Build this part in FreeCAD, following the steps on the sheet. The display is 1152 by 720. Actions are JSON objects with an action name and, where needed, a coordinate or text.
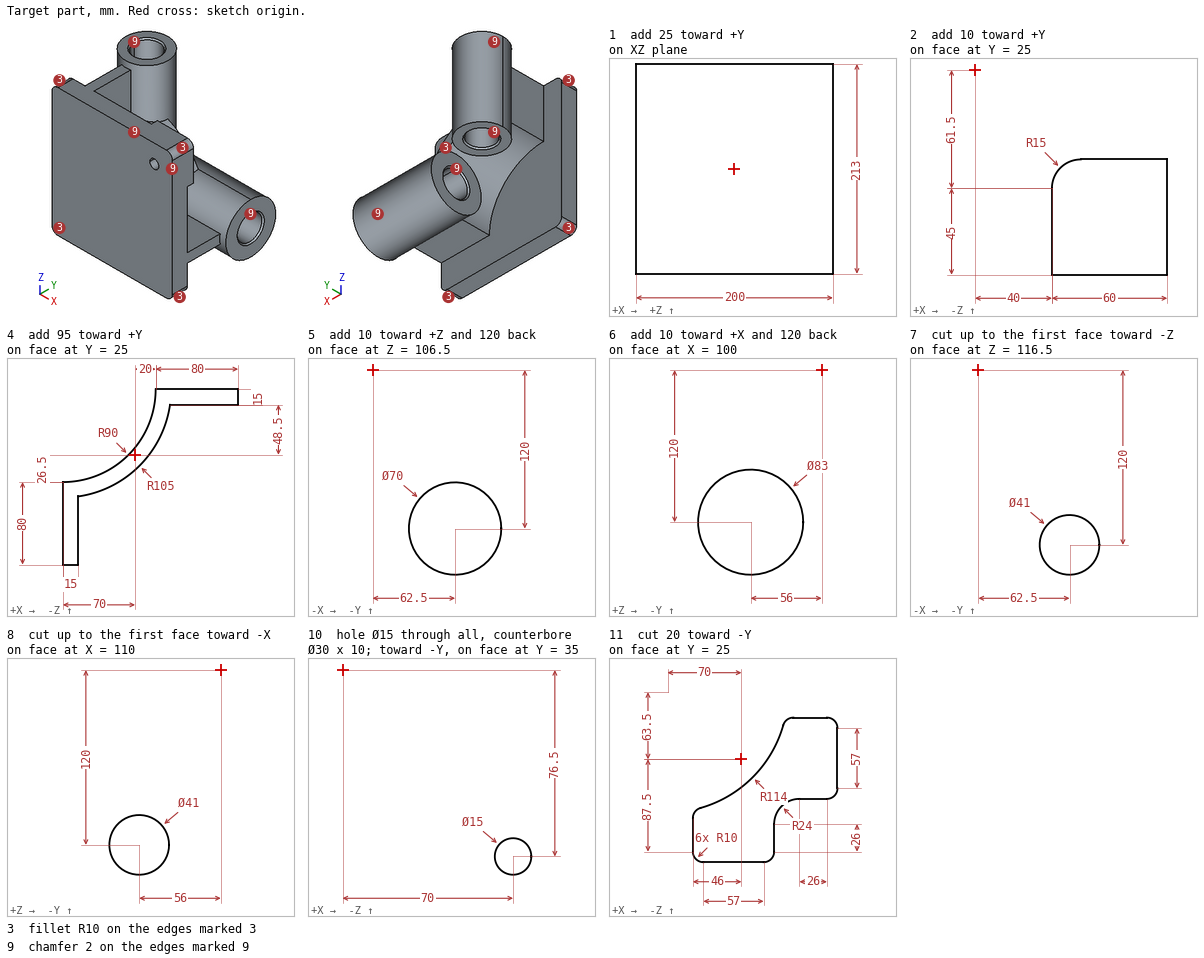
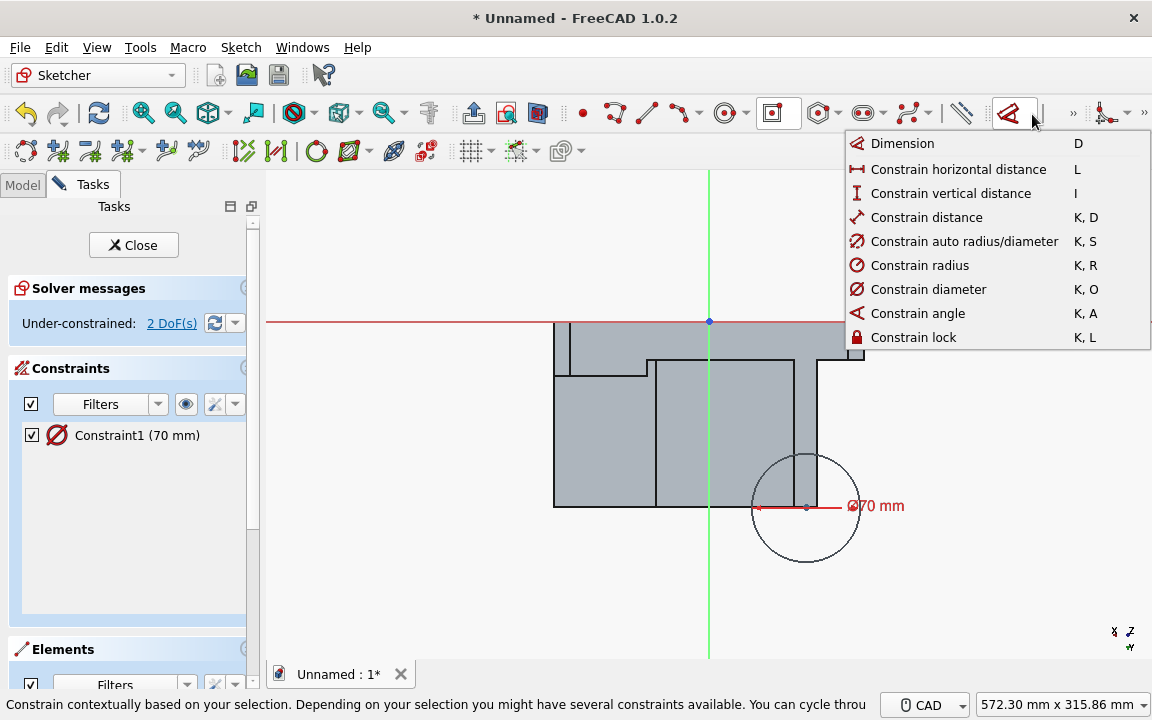
{"action": "left_click", "coordinate": [998, 193]}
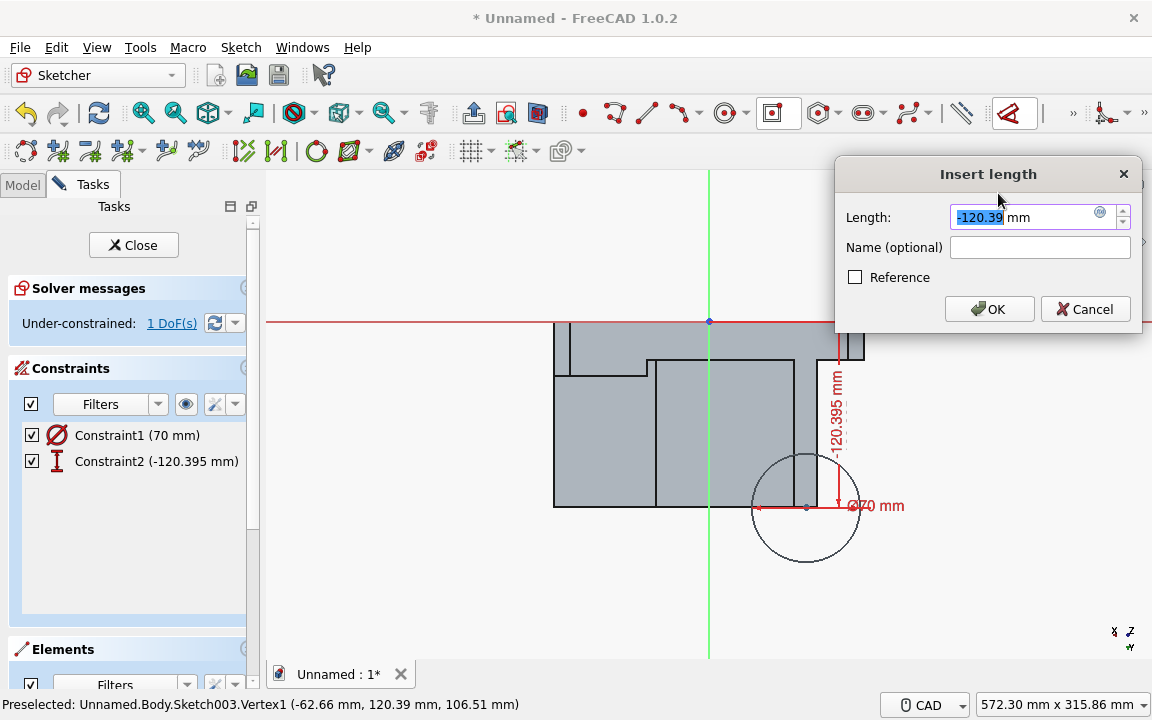
{"action": "type", "text": "-120"}
{"action": "key", "text": "Return"}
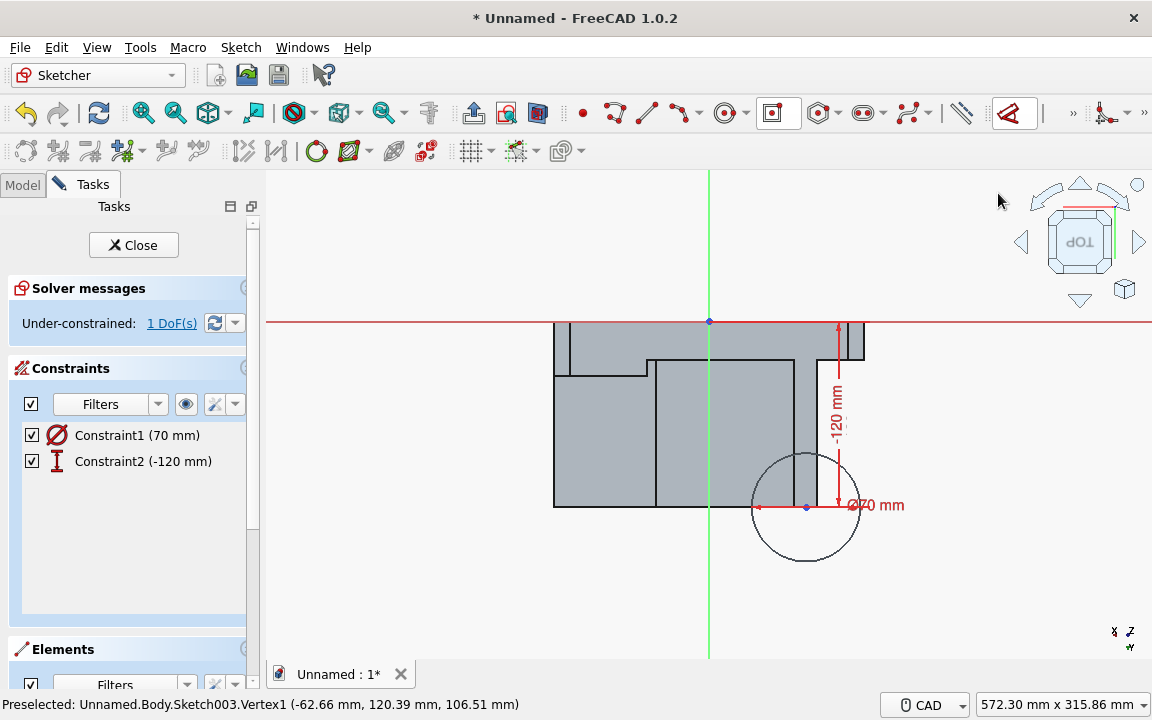
{"action": "left_click", "coordinate": [806, 507]}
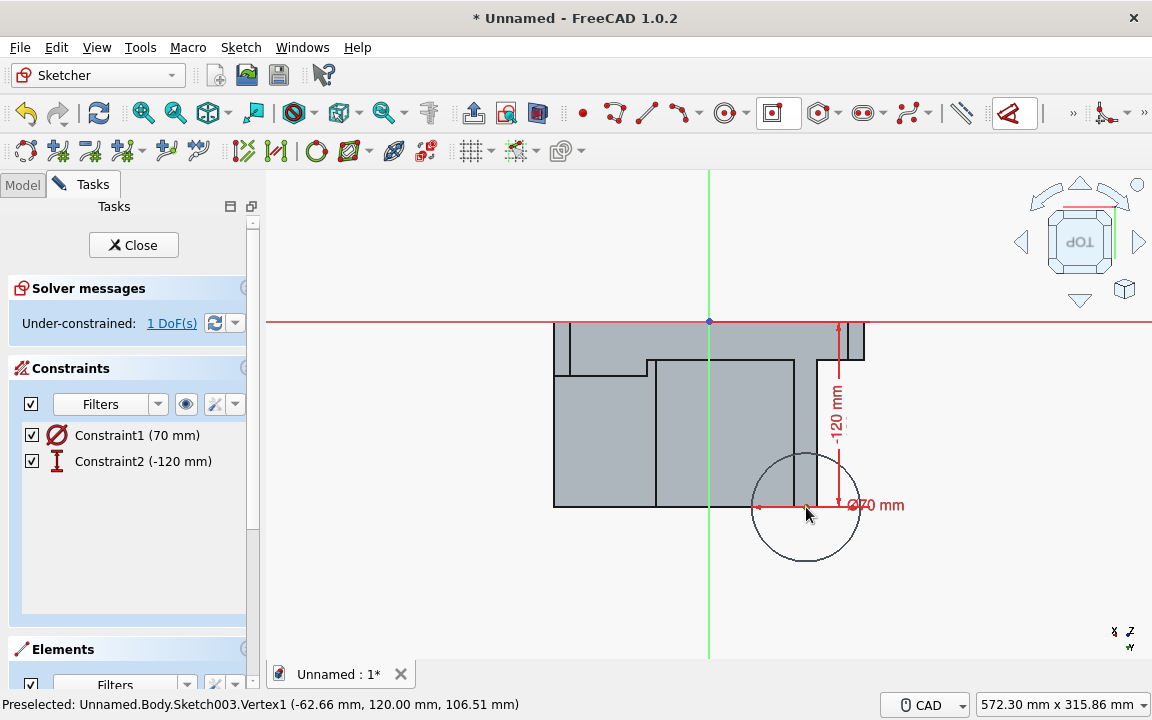
{"action": "left_click", "coordinate": [1032, 114]}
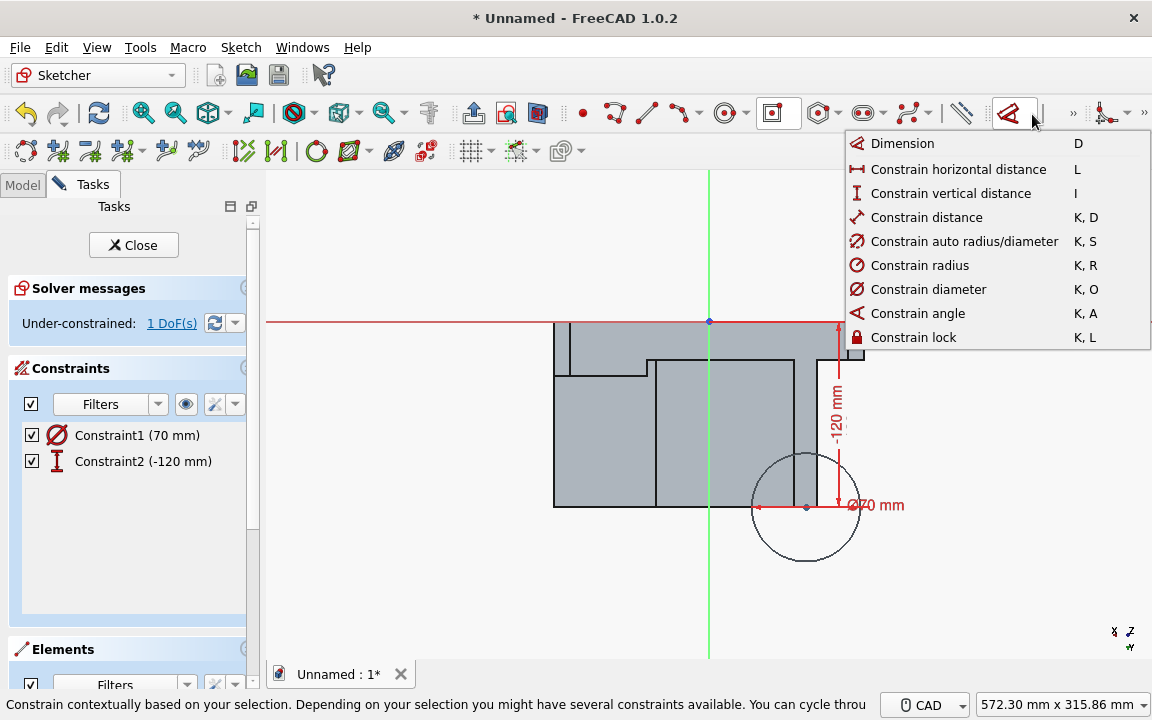
{"action": "left_click", "coordinate": [998, 169]}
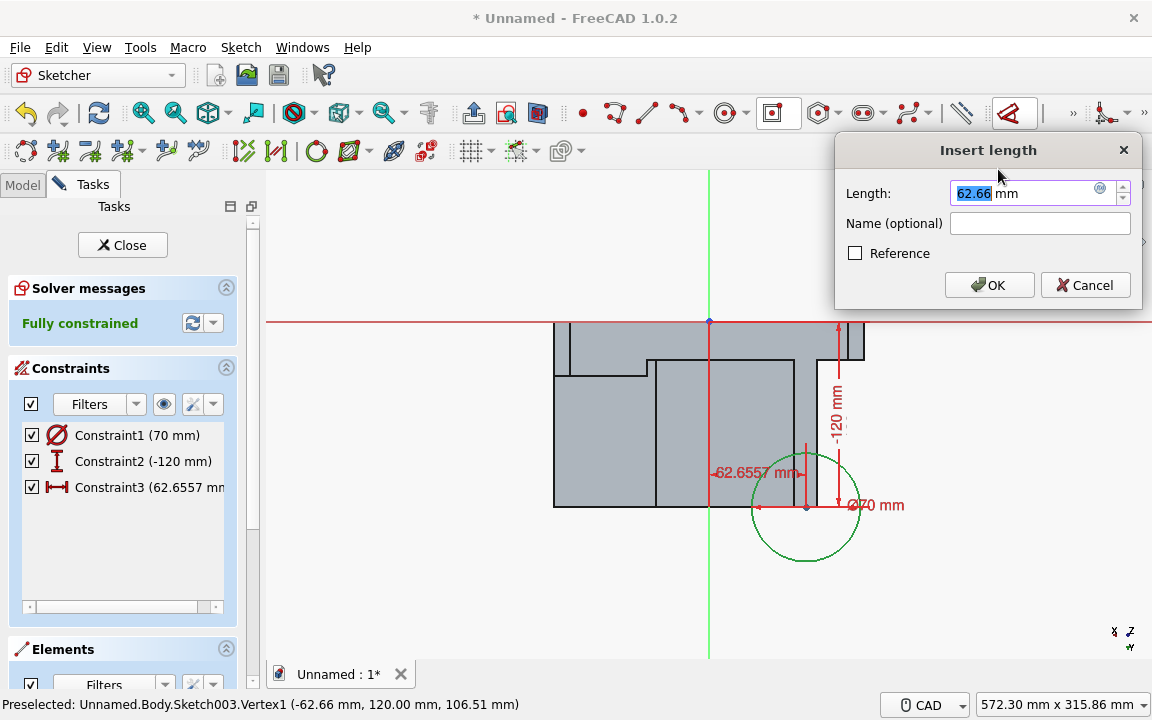
{"action": "type", "text": "62.5"}
{"action": "key", "text": "Return"}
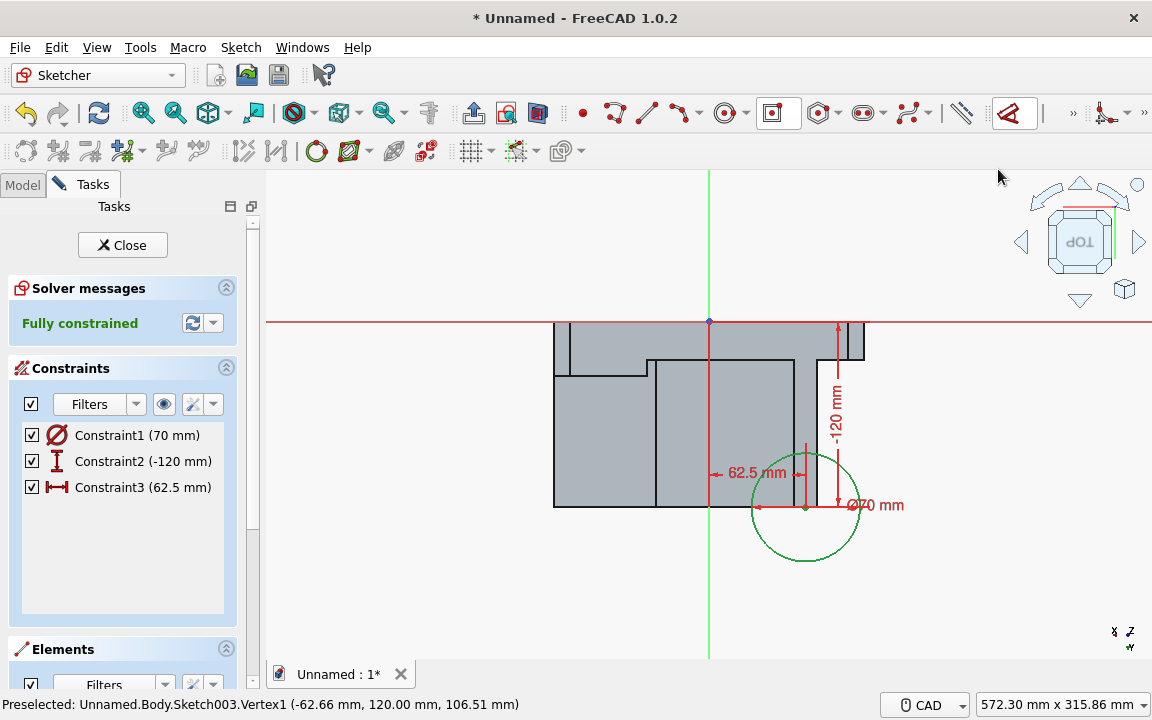
{"action": "left_click", "coordinate": [123, 245]}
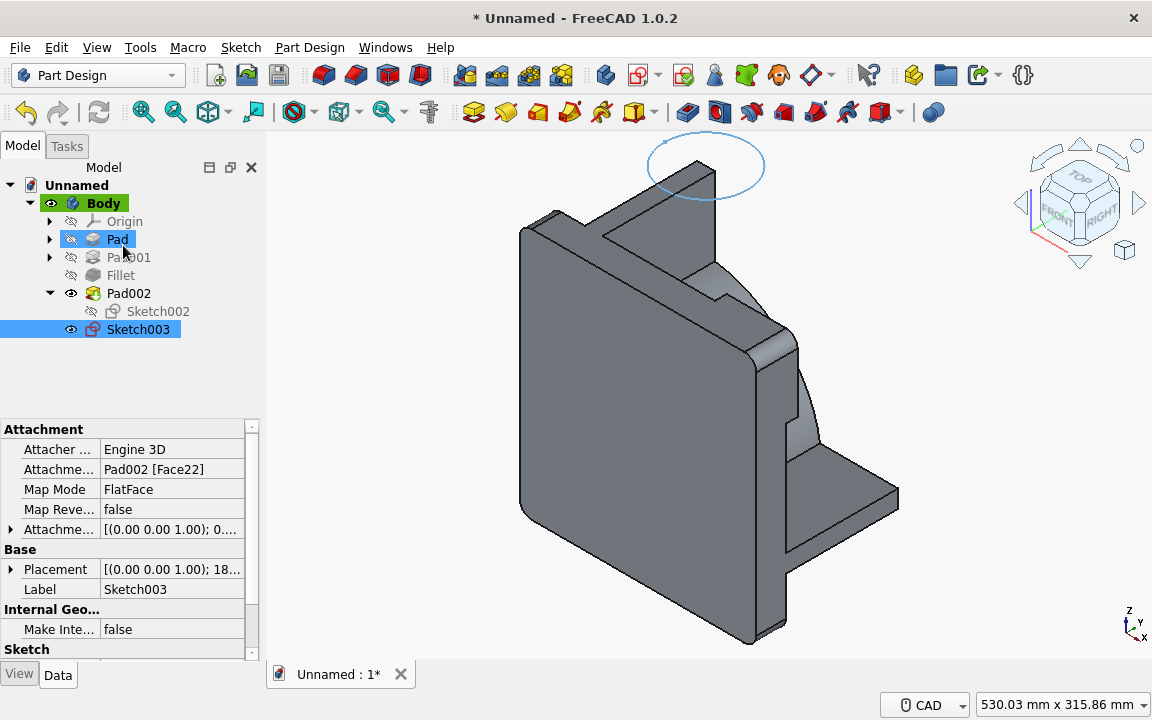
{"action": "left_click", "coordinate": [474, 112]}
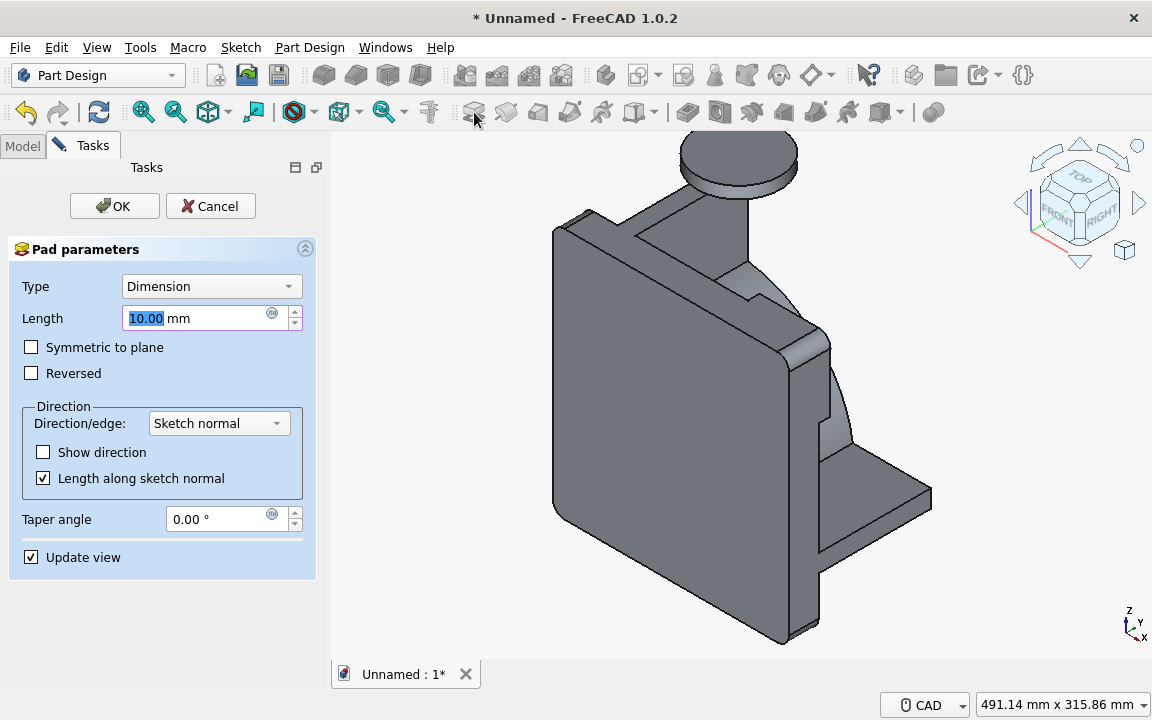
{"action": "left_click", "coordinate": [212, 286]}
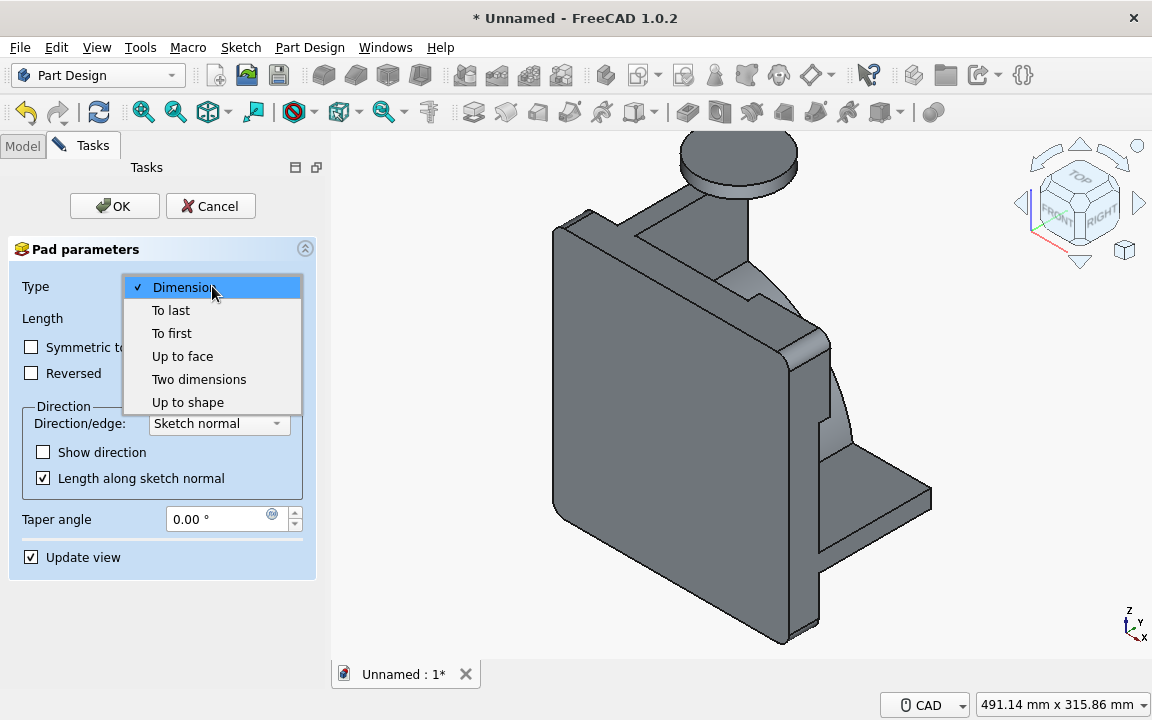
{"action": "left_click", "coordinate": [212, 380]}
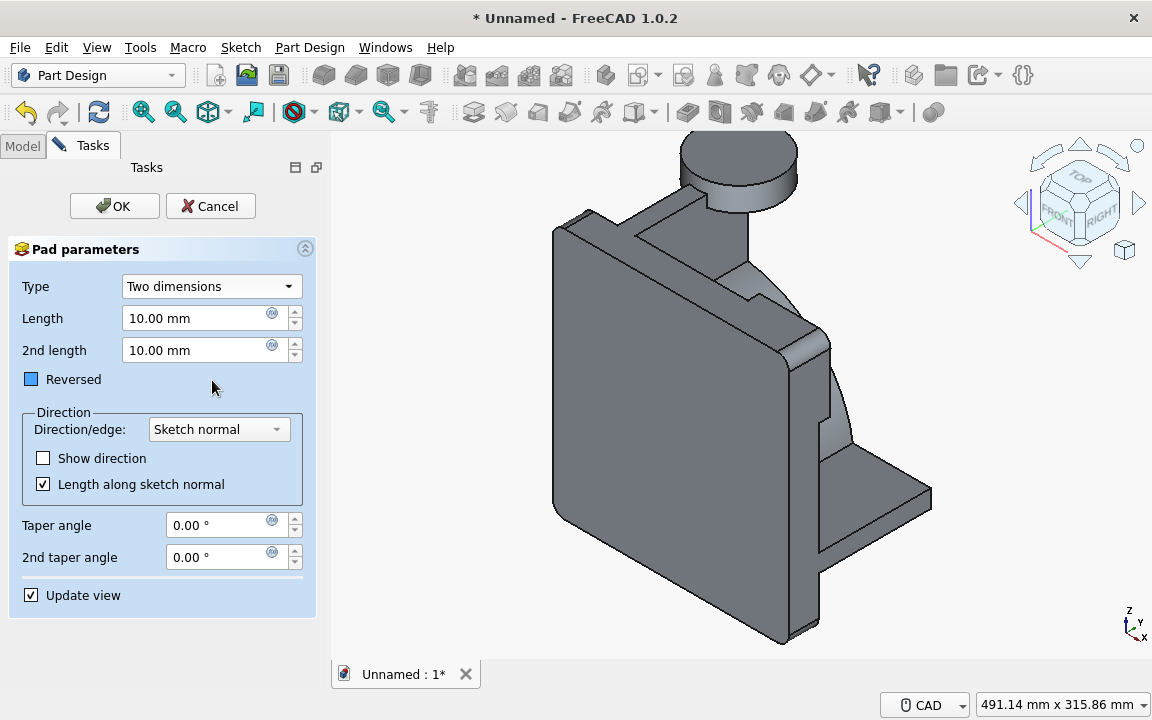
{"action": "triple_click", "coordinate": [204, 318]}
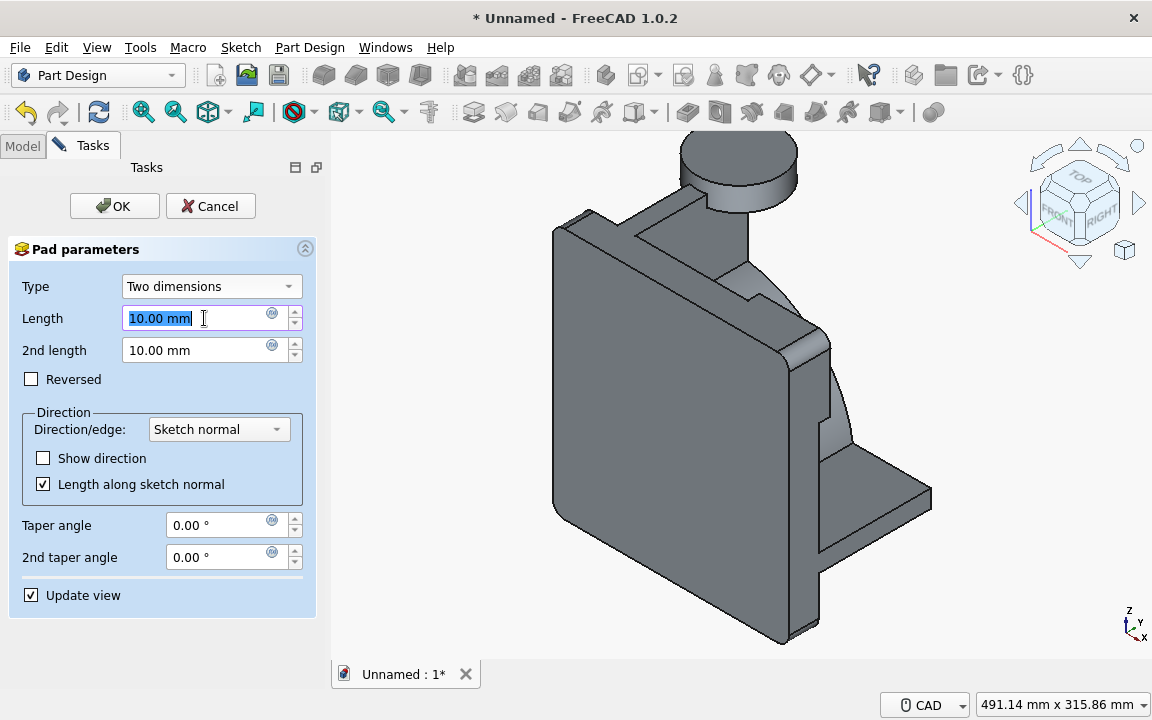
{"action": "type", "text": "10"}
{"action": "key", "text": "Tab"}